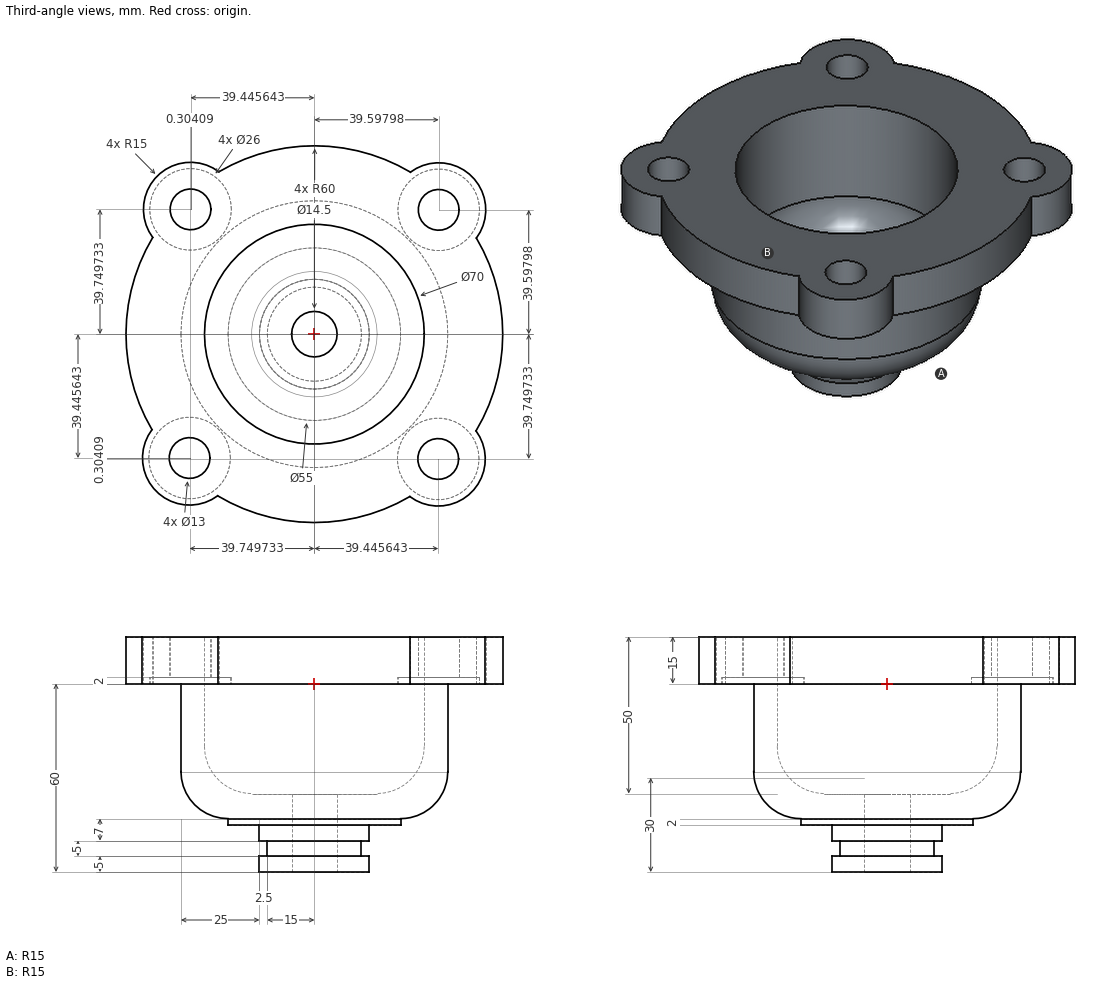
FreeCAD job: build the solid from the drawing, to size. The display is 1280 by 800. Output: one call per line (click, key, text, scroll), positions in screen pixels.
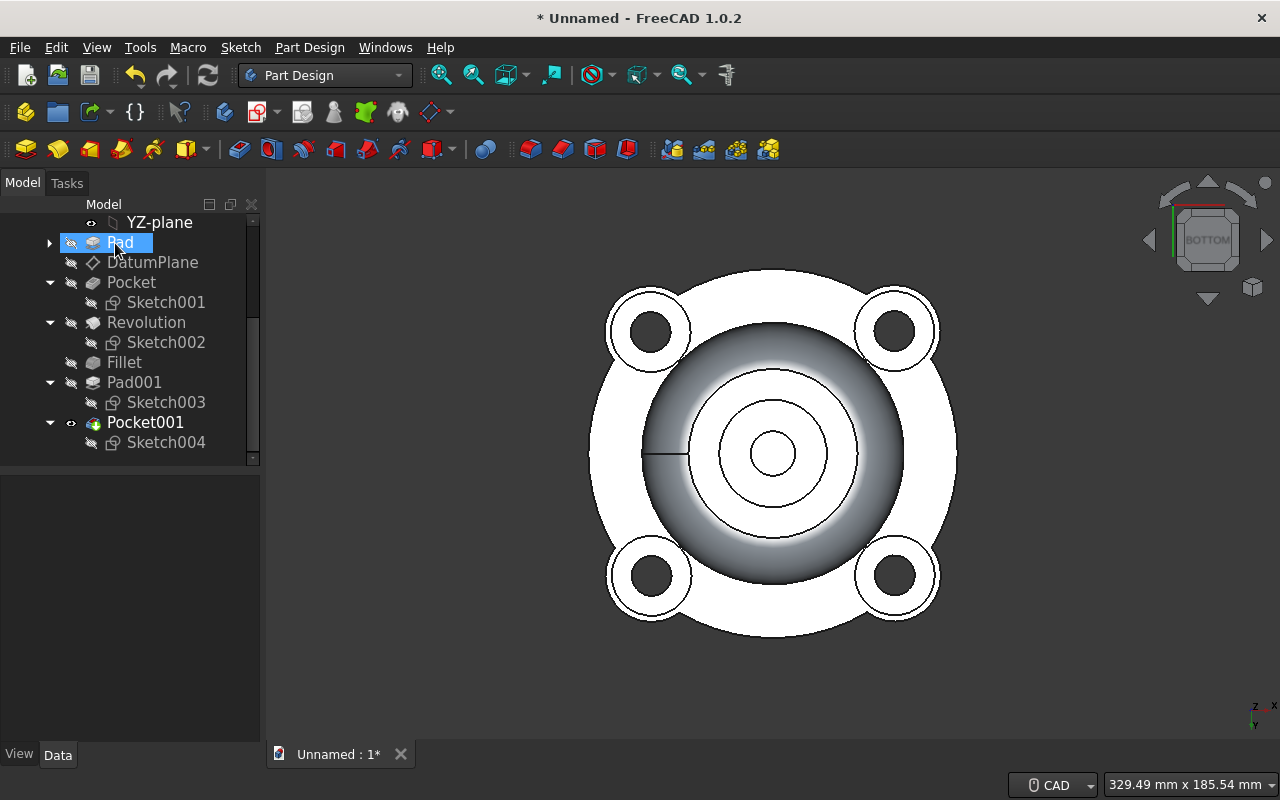
key(0)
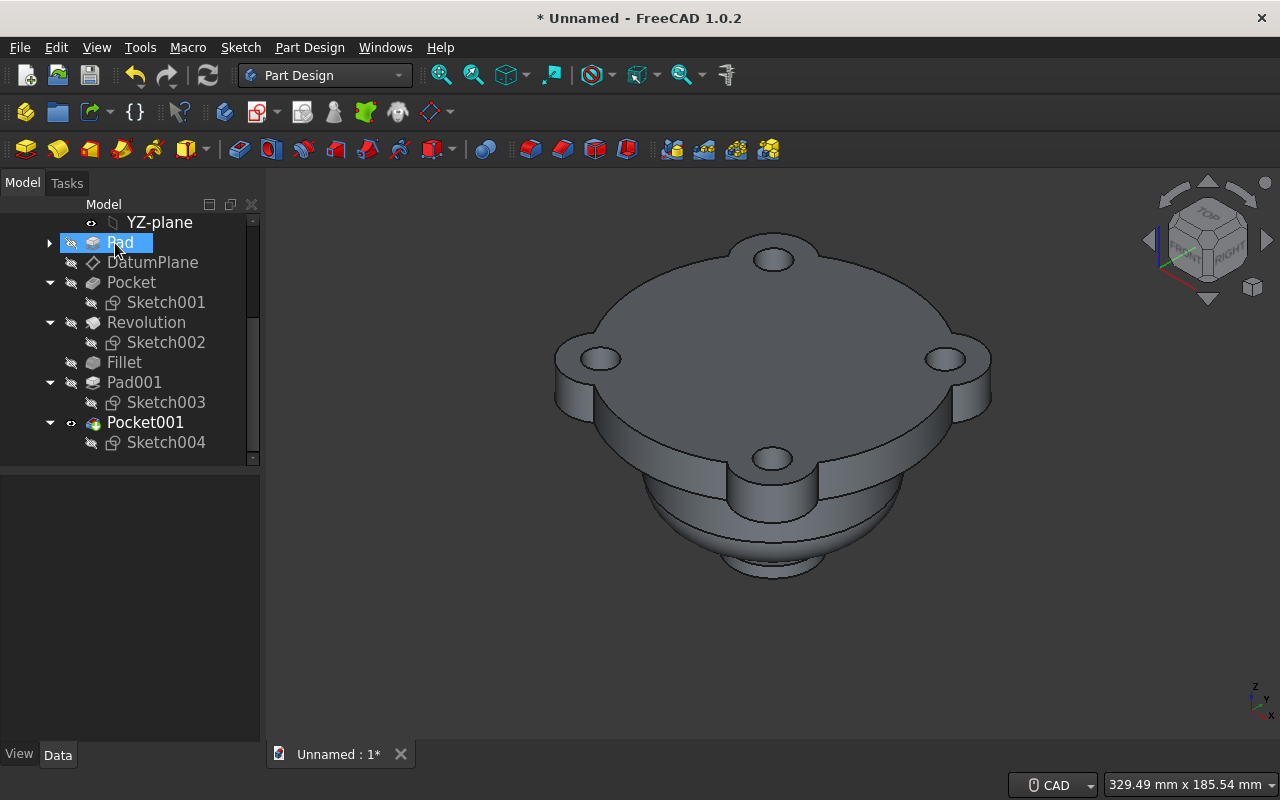
click(773, 358)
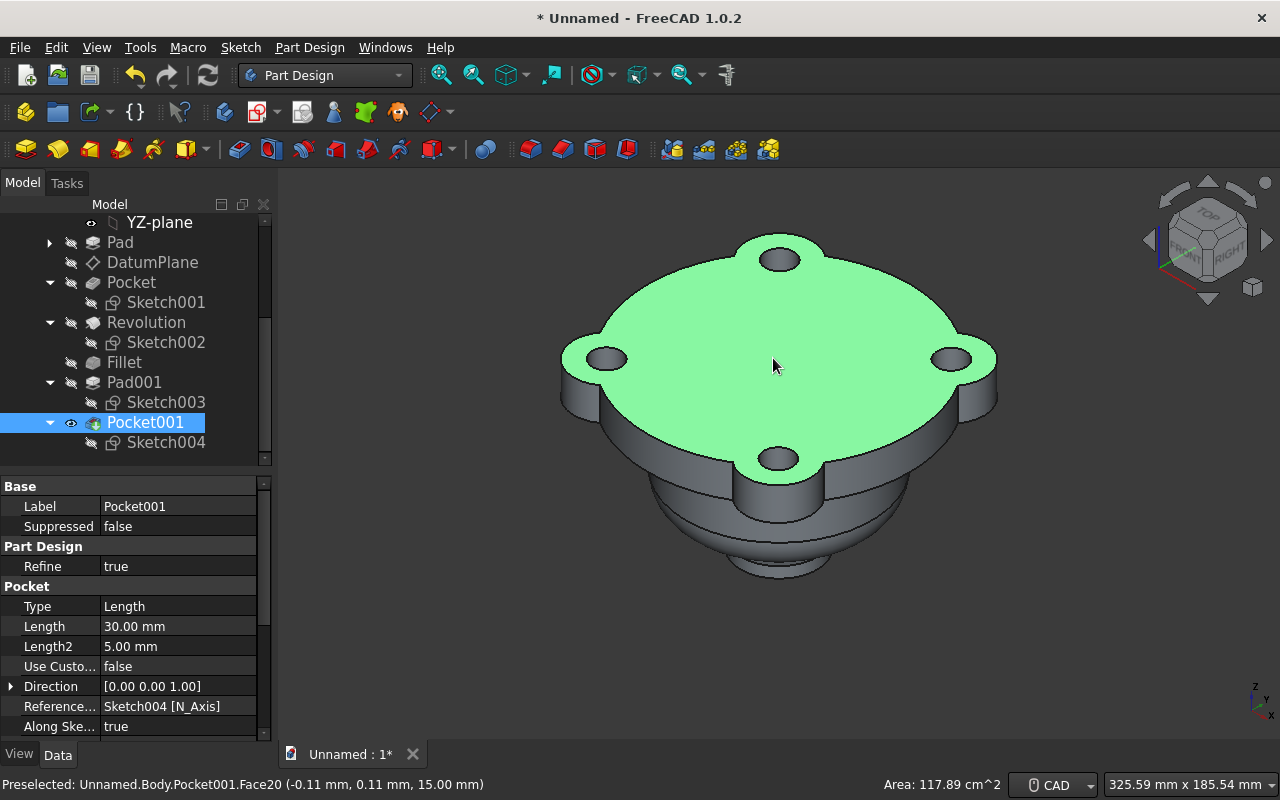
click(258, 112)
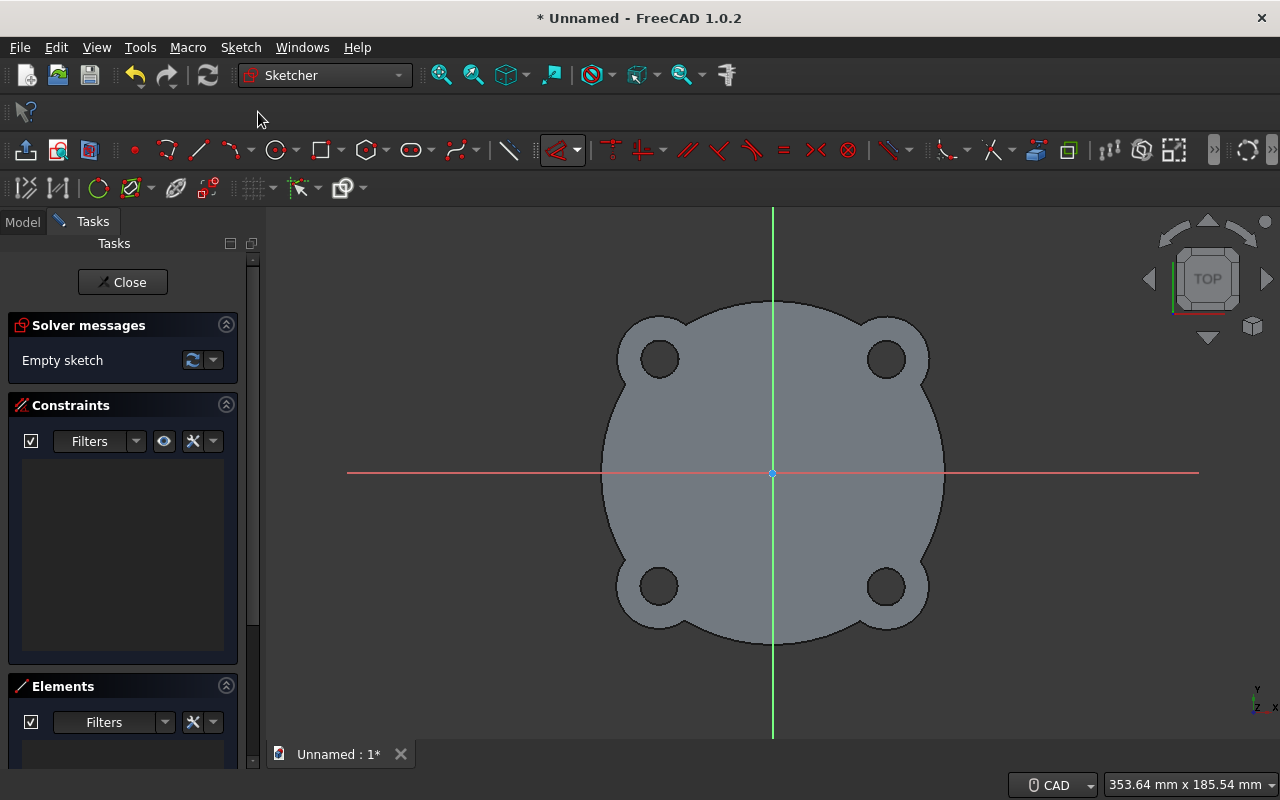
scroll(856, 473, up, 3)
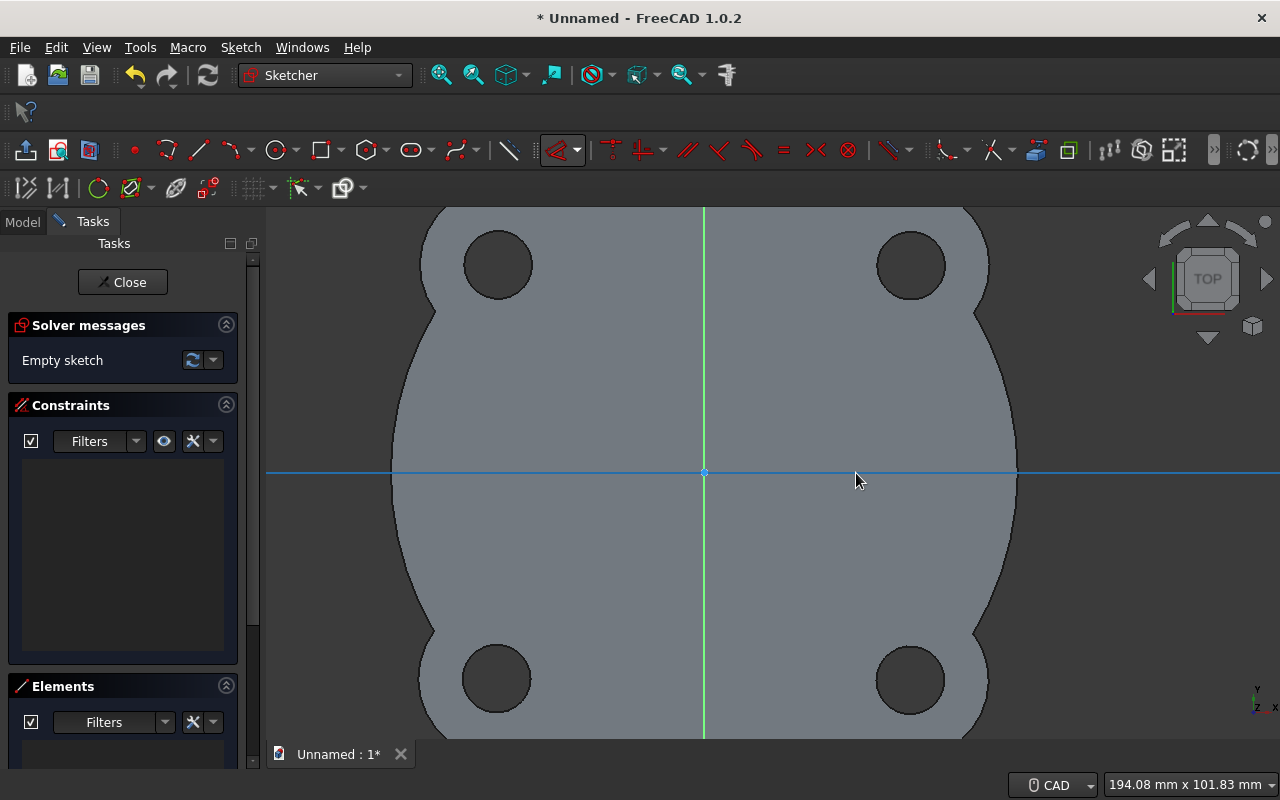
key(g)
key(c)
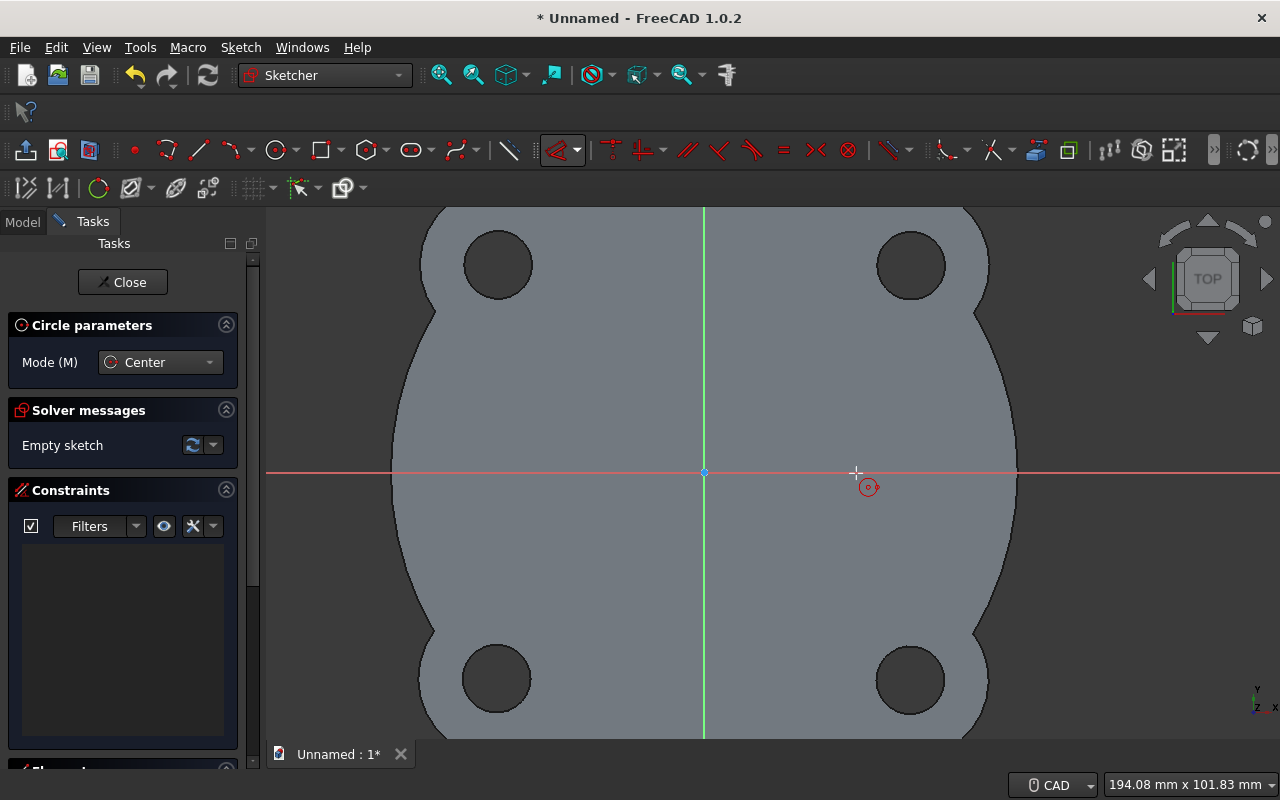
click(704, 473)
move(834, 343)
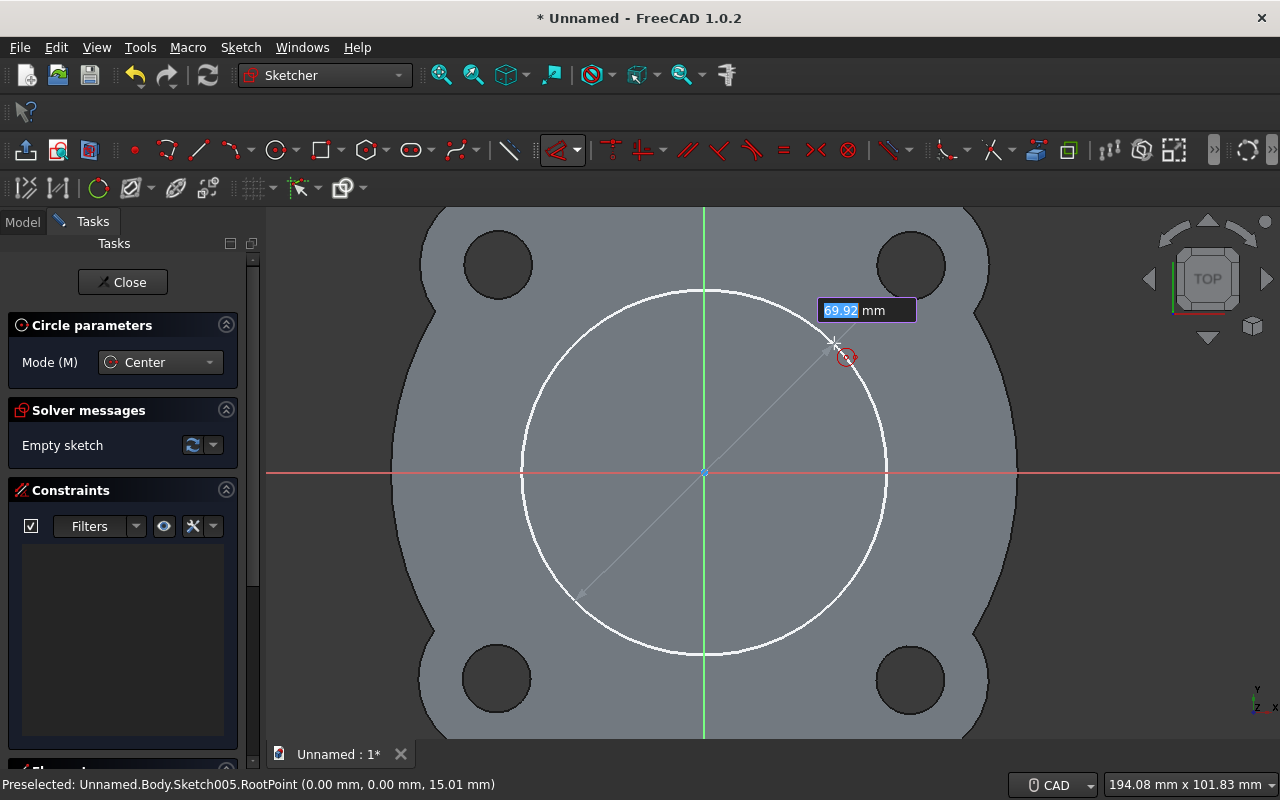
text(70)
key(Return)
key(Escape)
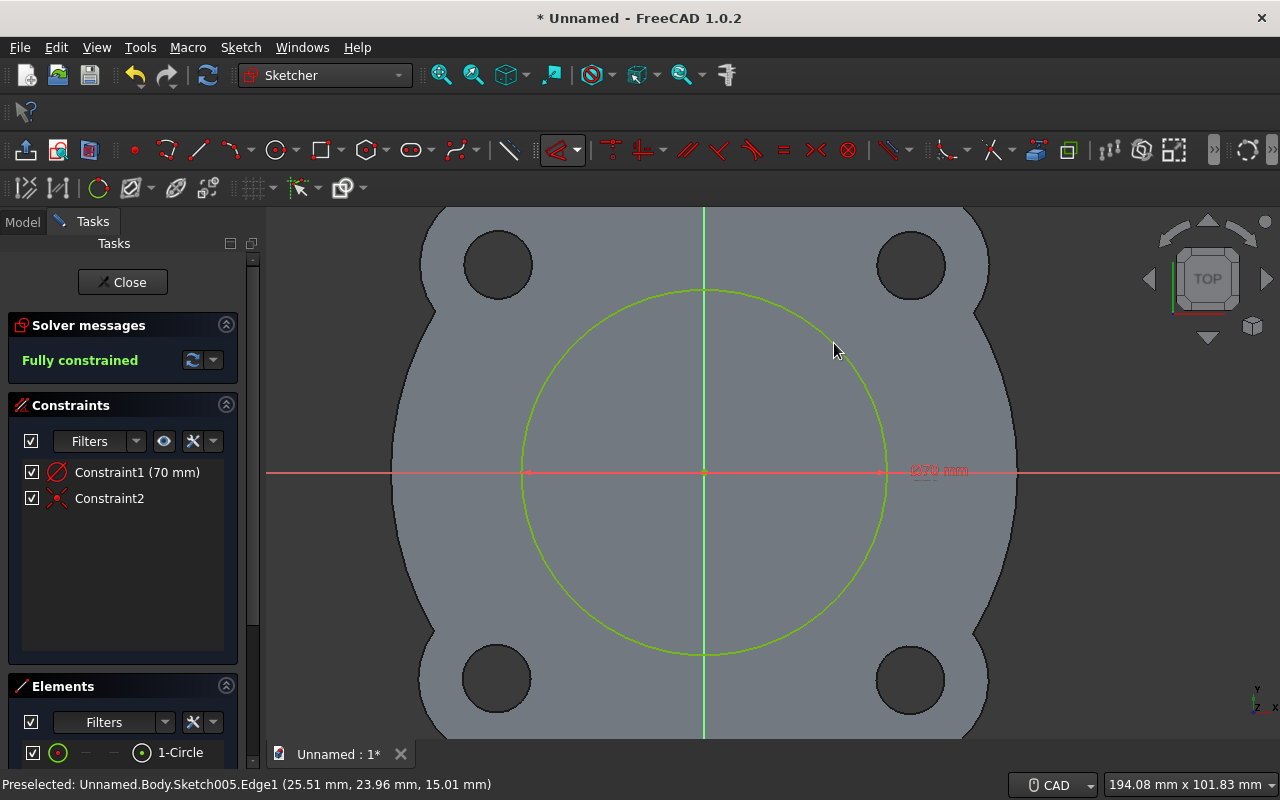
click(123, 282)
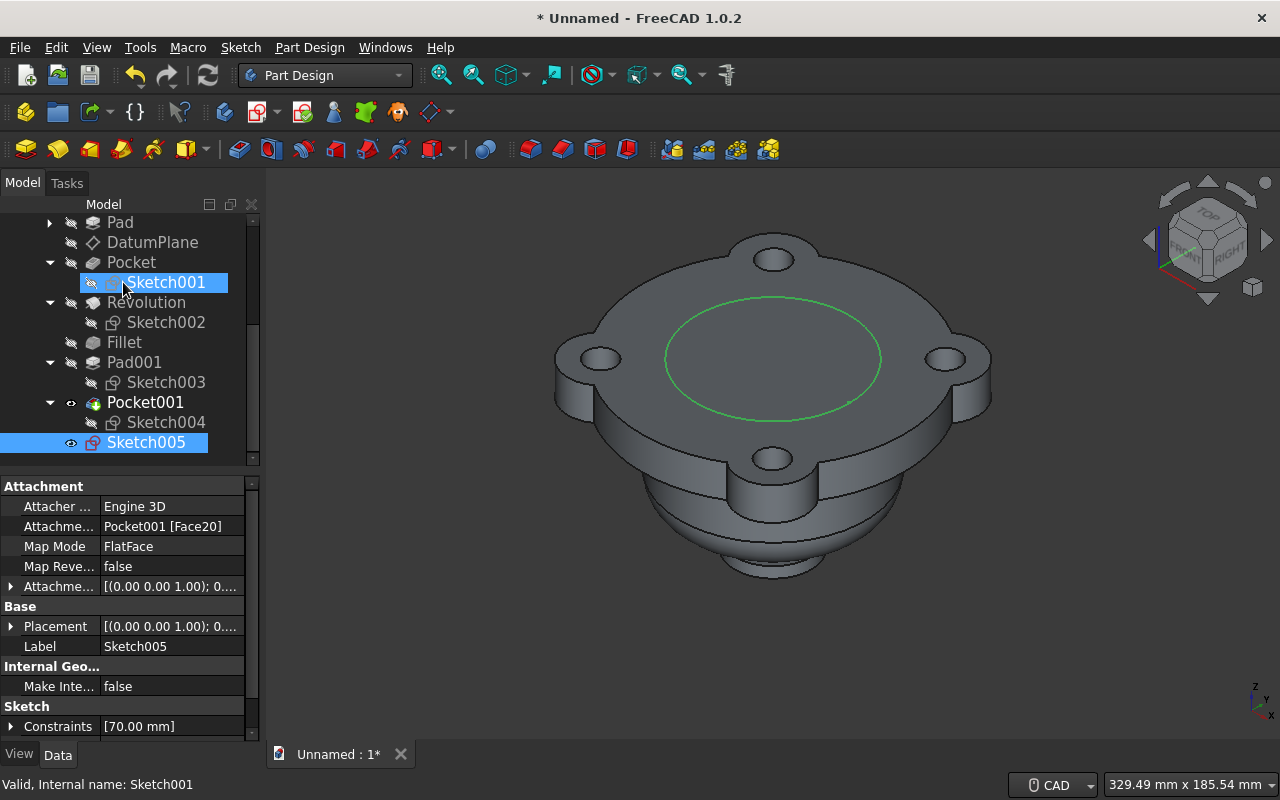
click(240, 150)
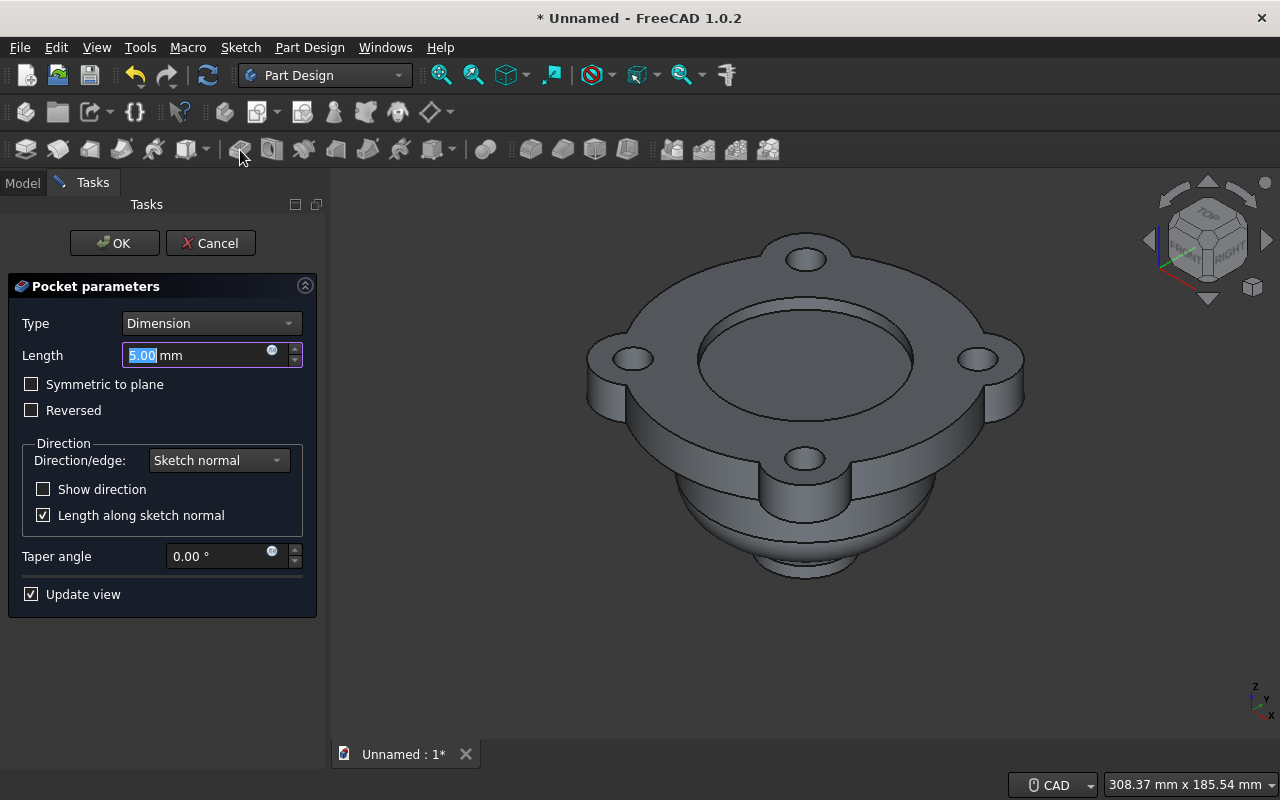
text(50)
key(Tab)